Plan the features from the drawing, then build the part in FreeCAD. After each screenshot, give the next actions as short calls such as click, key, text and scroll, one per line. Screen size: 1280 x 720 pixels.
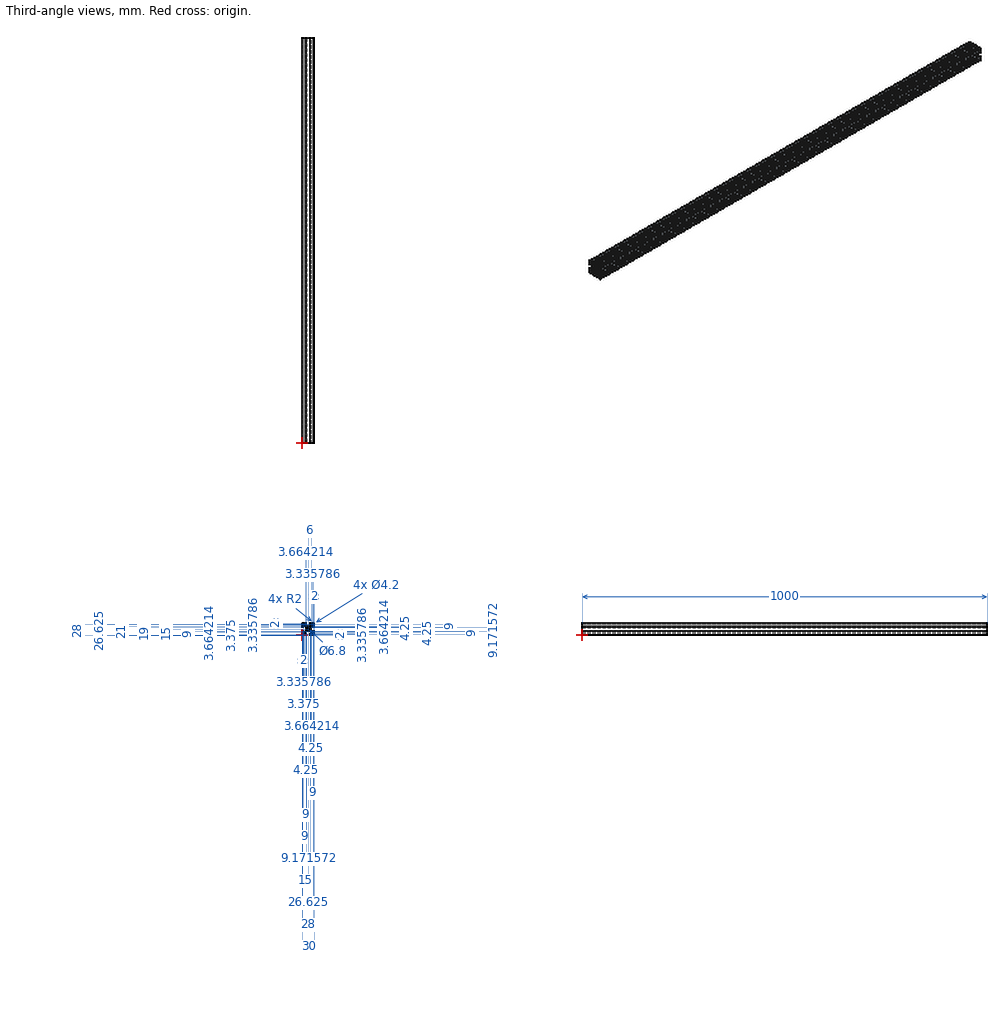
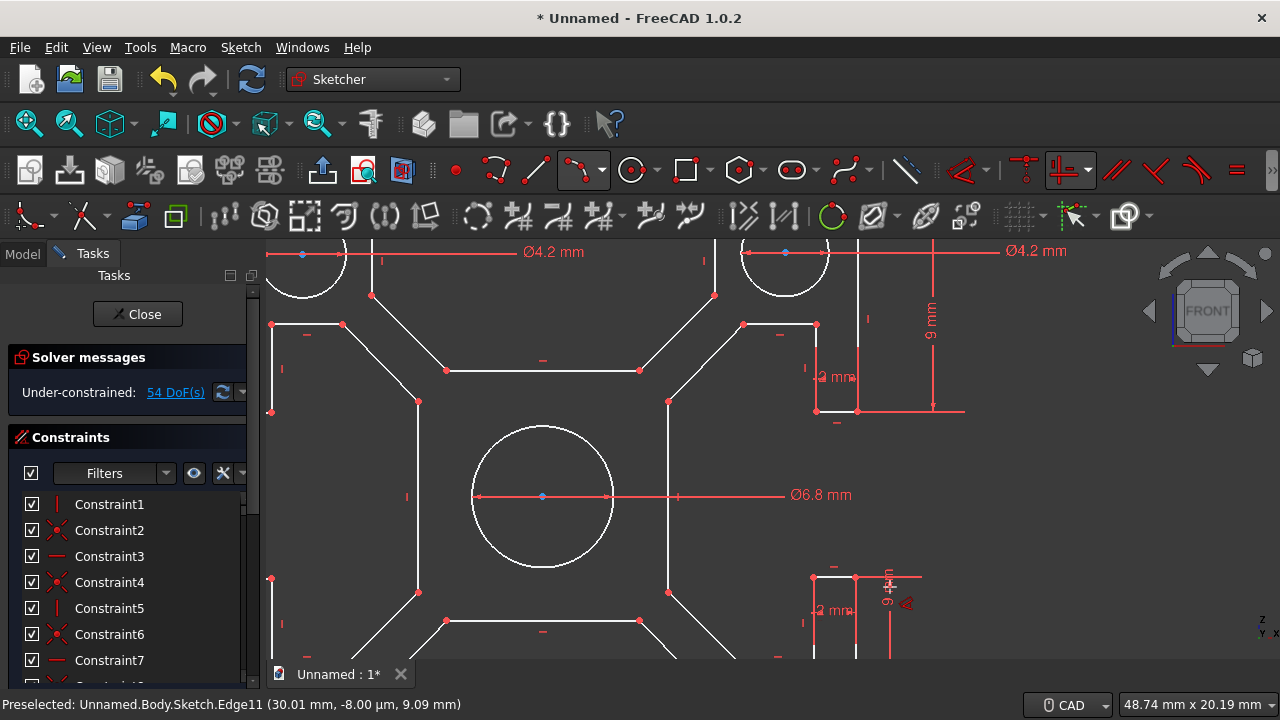
scroll(836, 412, down, 4)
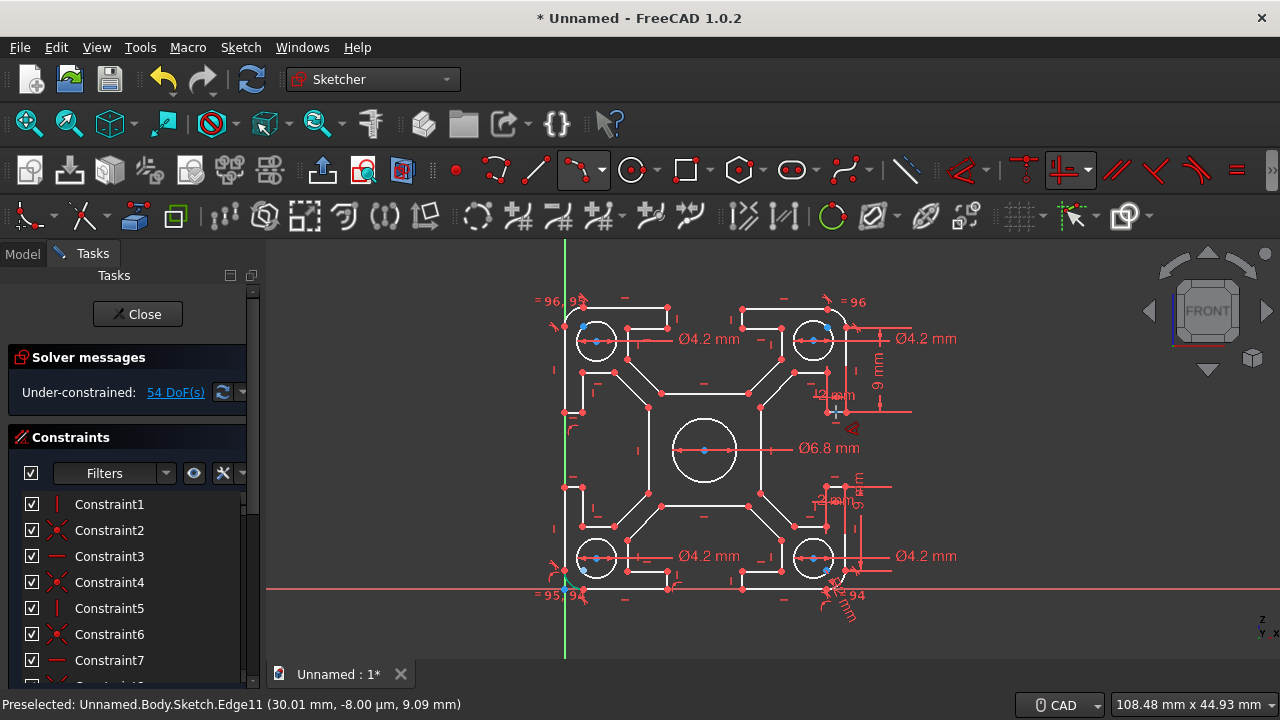
click(801, 589)
click(784, 623)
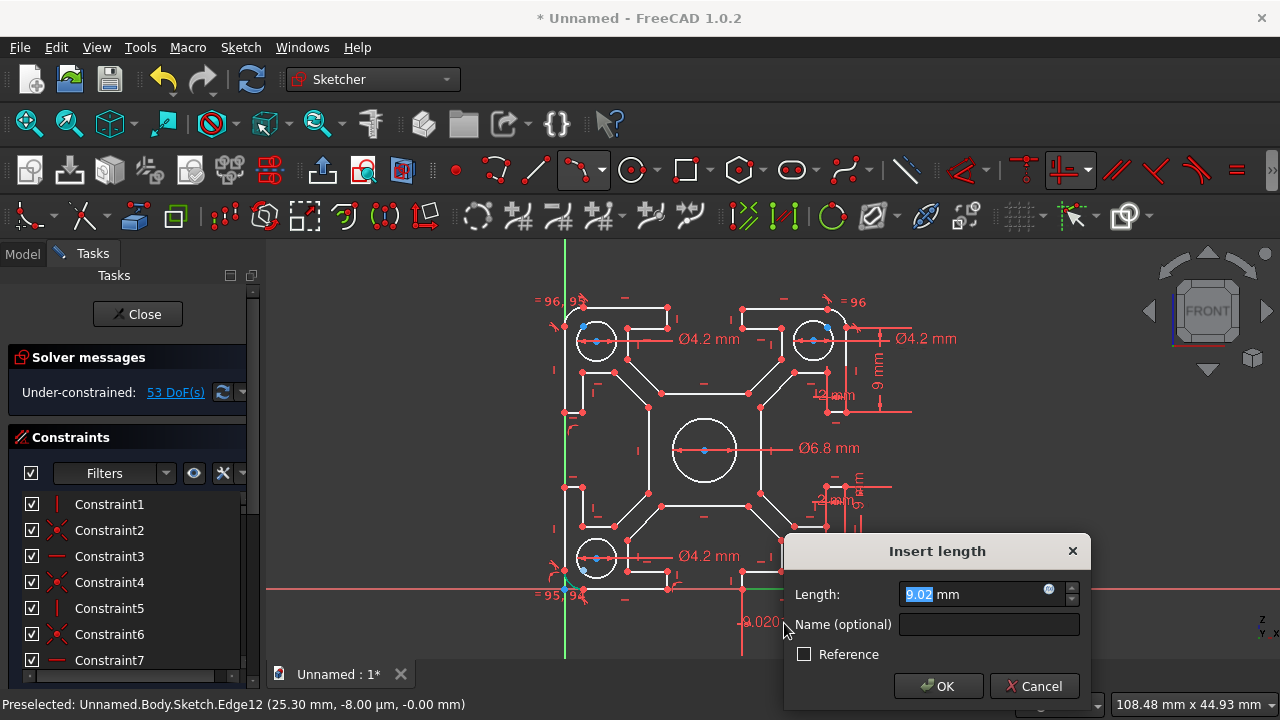
text(9)
key(Return)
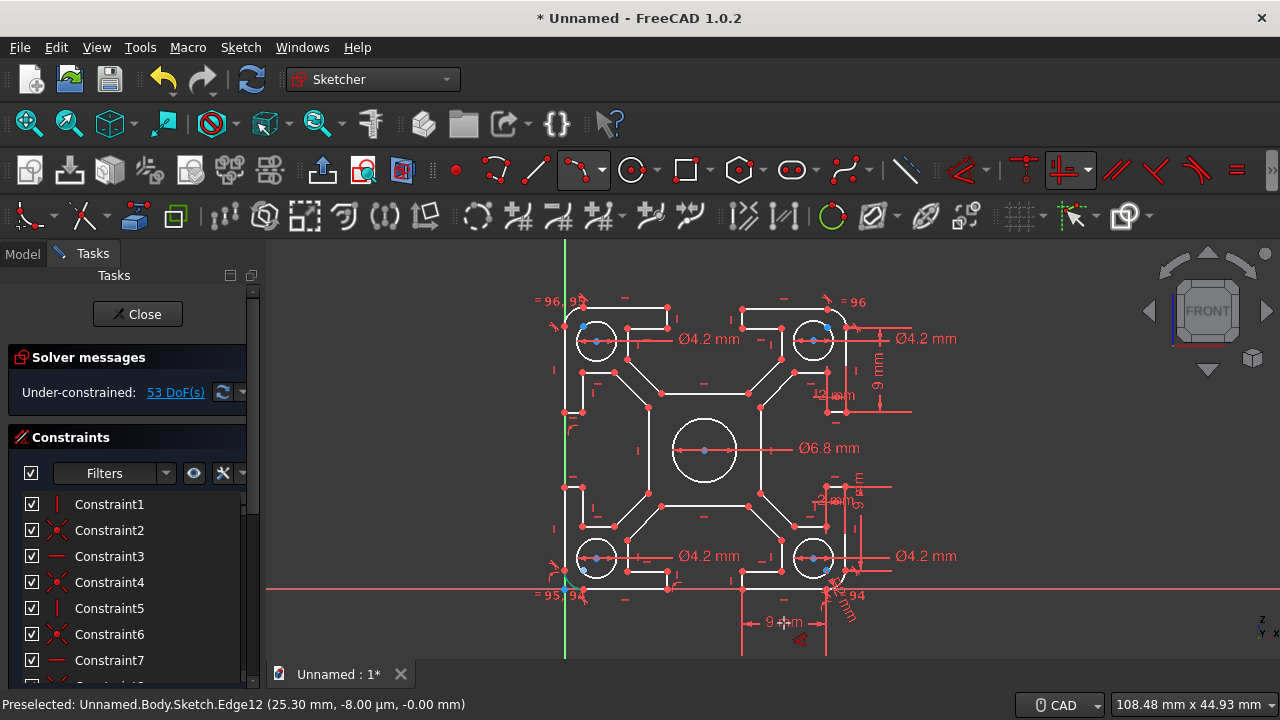
scroll(742, 581, up, 4)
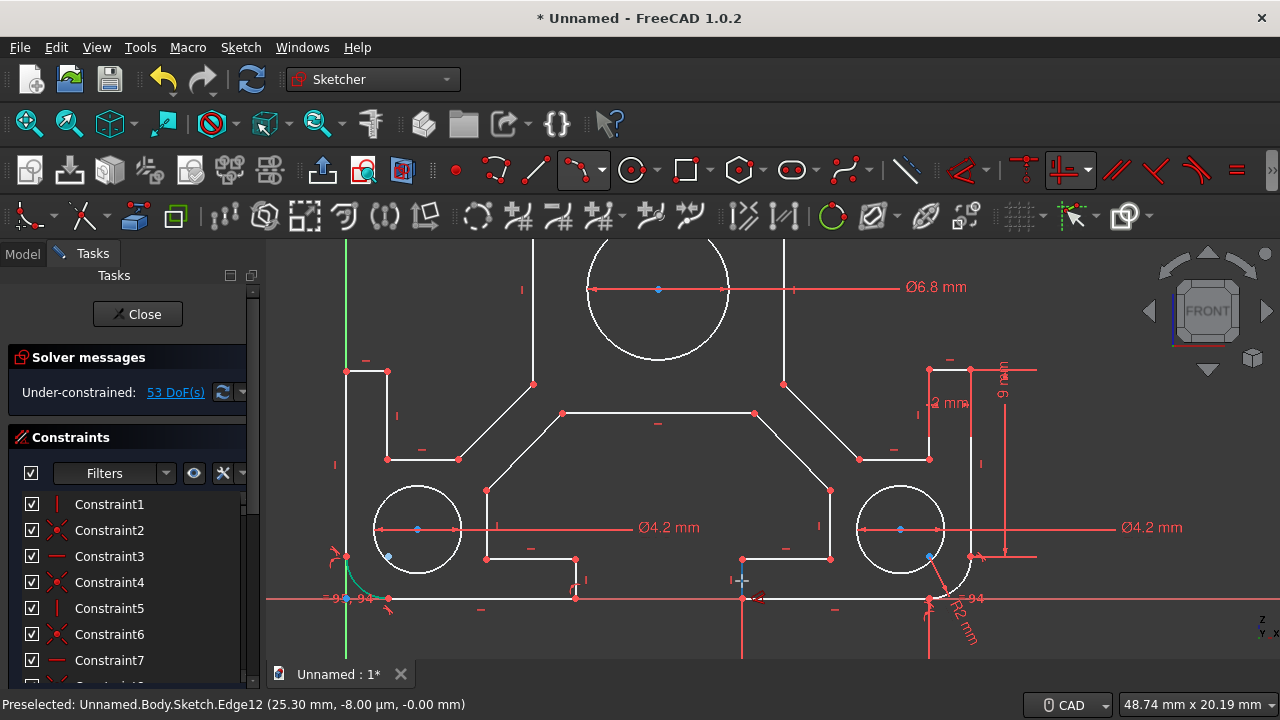
click(742, 579)
click(776, 579)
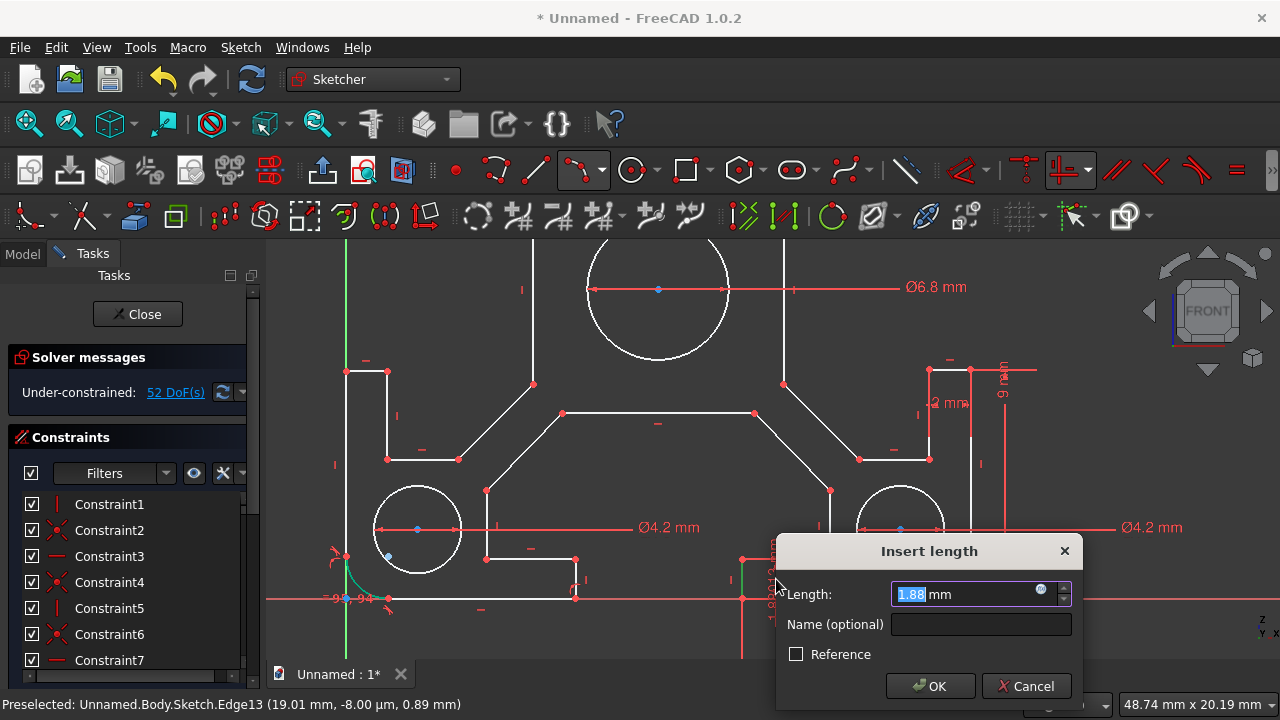
text(2)
key(Return)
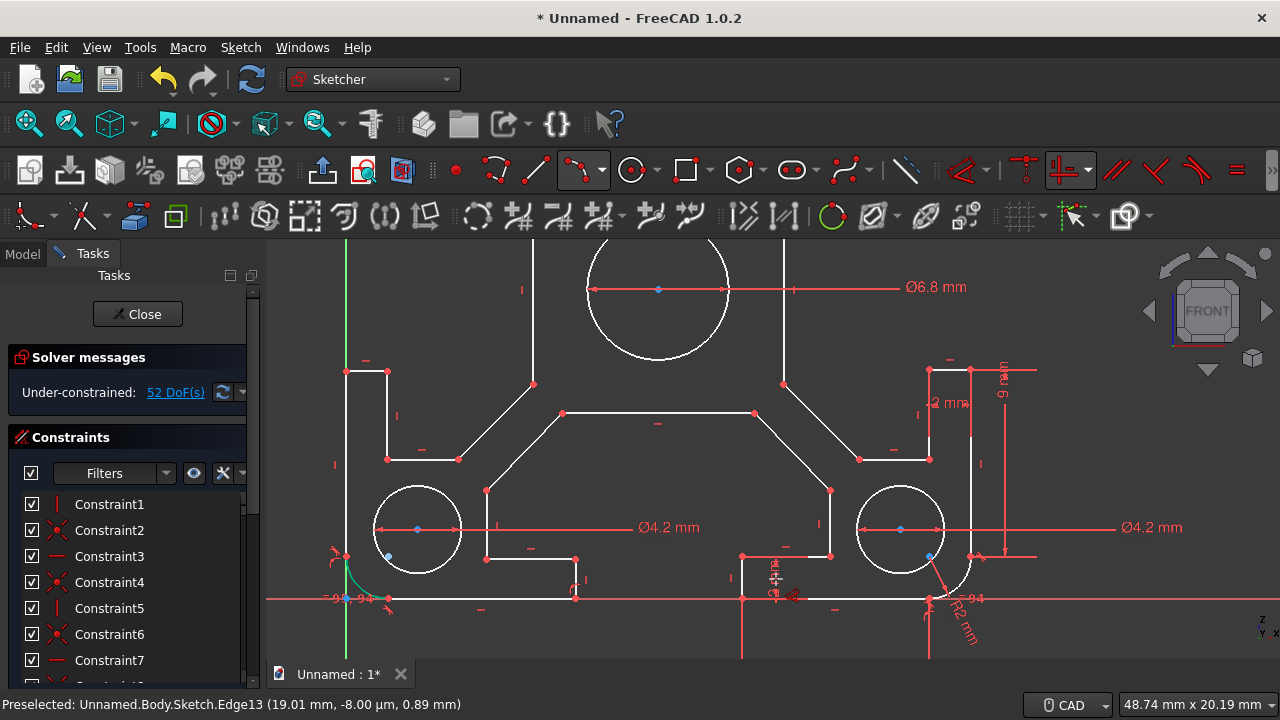
click(576, 571)
click(542, 579)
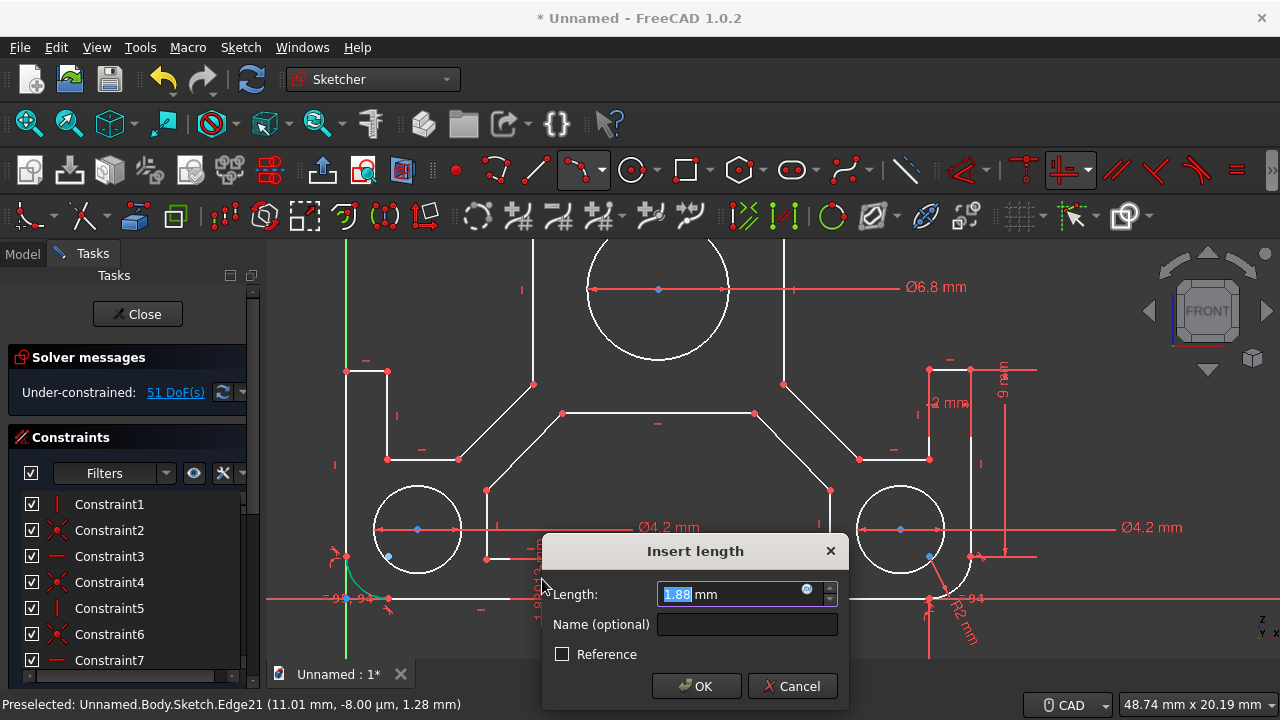
text(2)
key(Return)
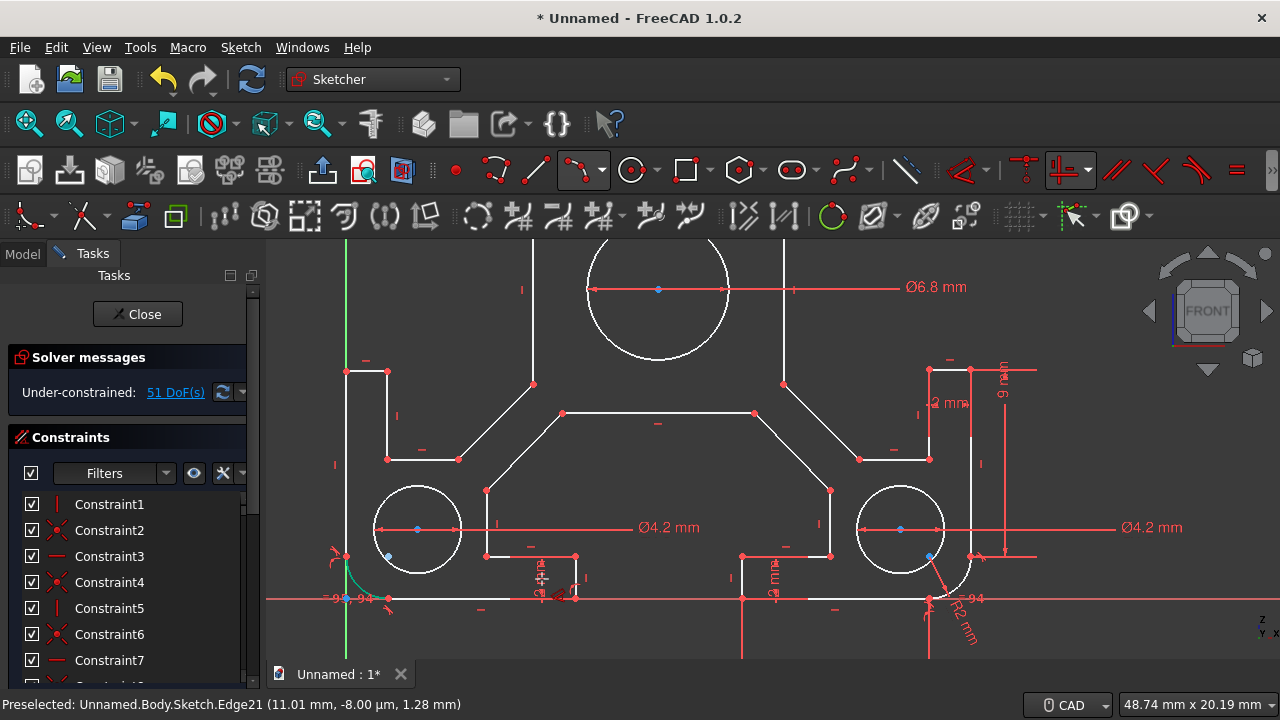
click(519, 599)
click(439, 541)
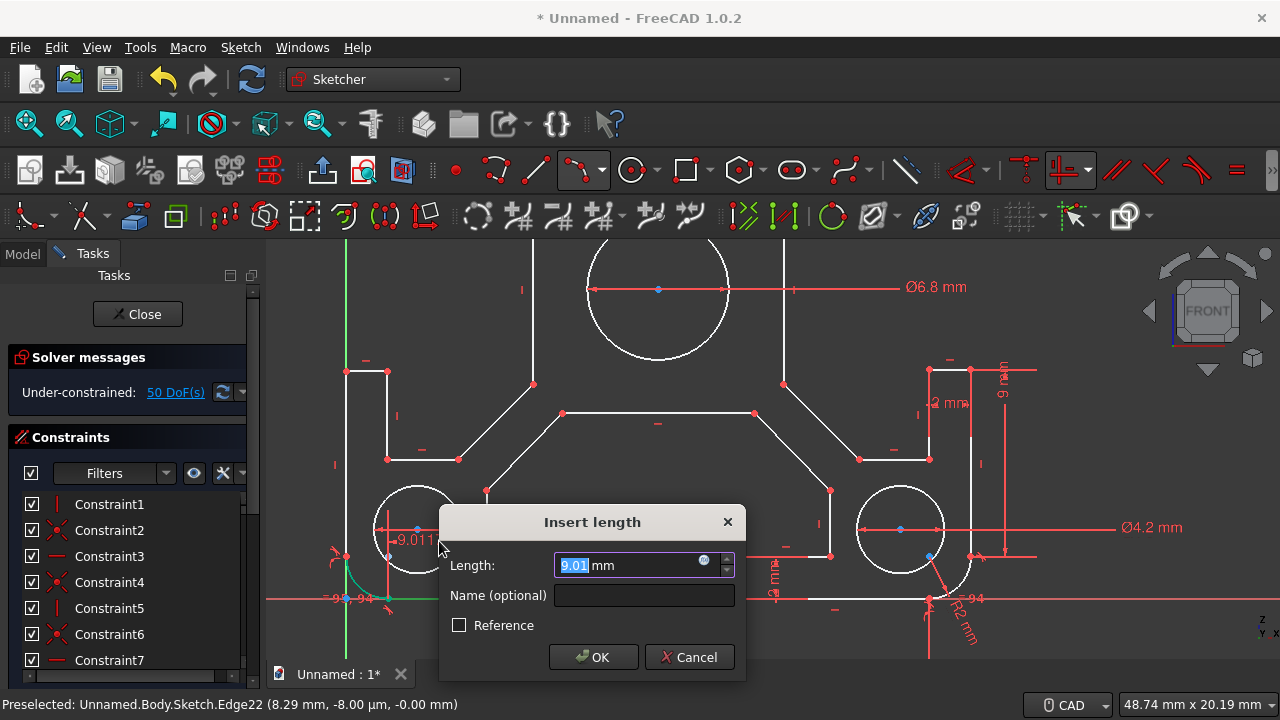
text(9)
key(Return)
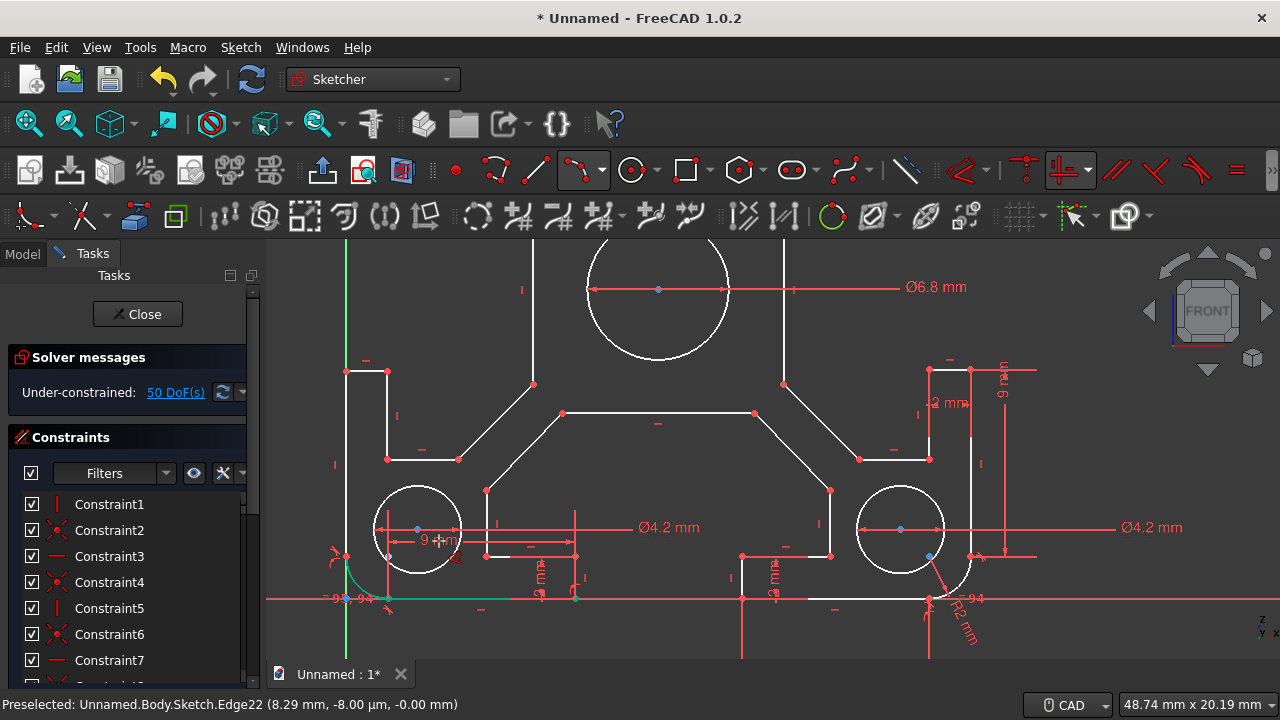
click(346, 501)
click(312, 464)